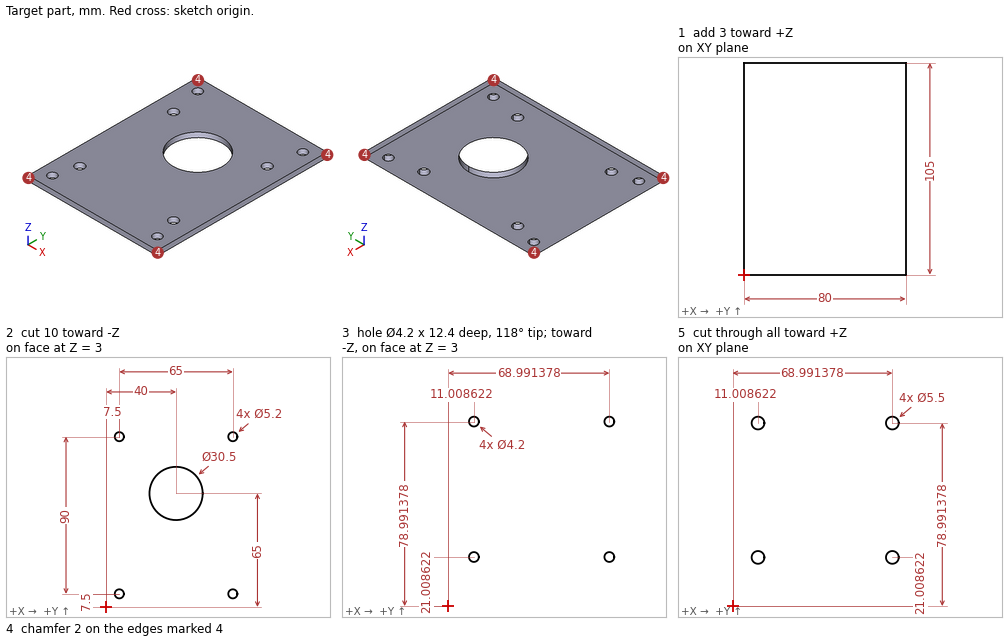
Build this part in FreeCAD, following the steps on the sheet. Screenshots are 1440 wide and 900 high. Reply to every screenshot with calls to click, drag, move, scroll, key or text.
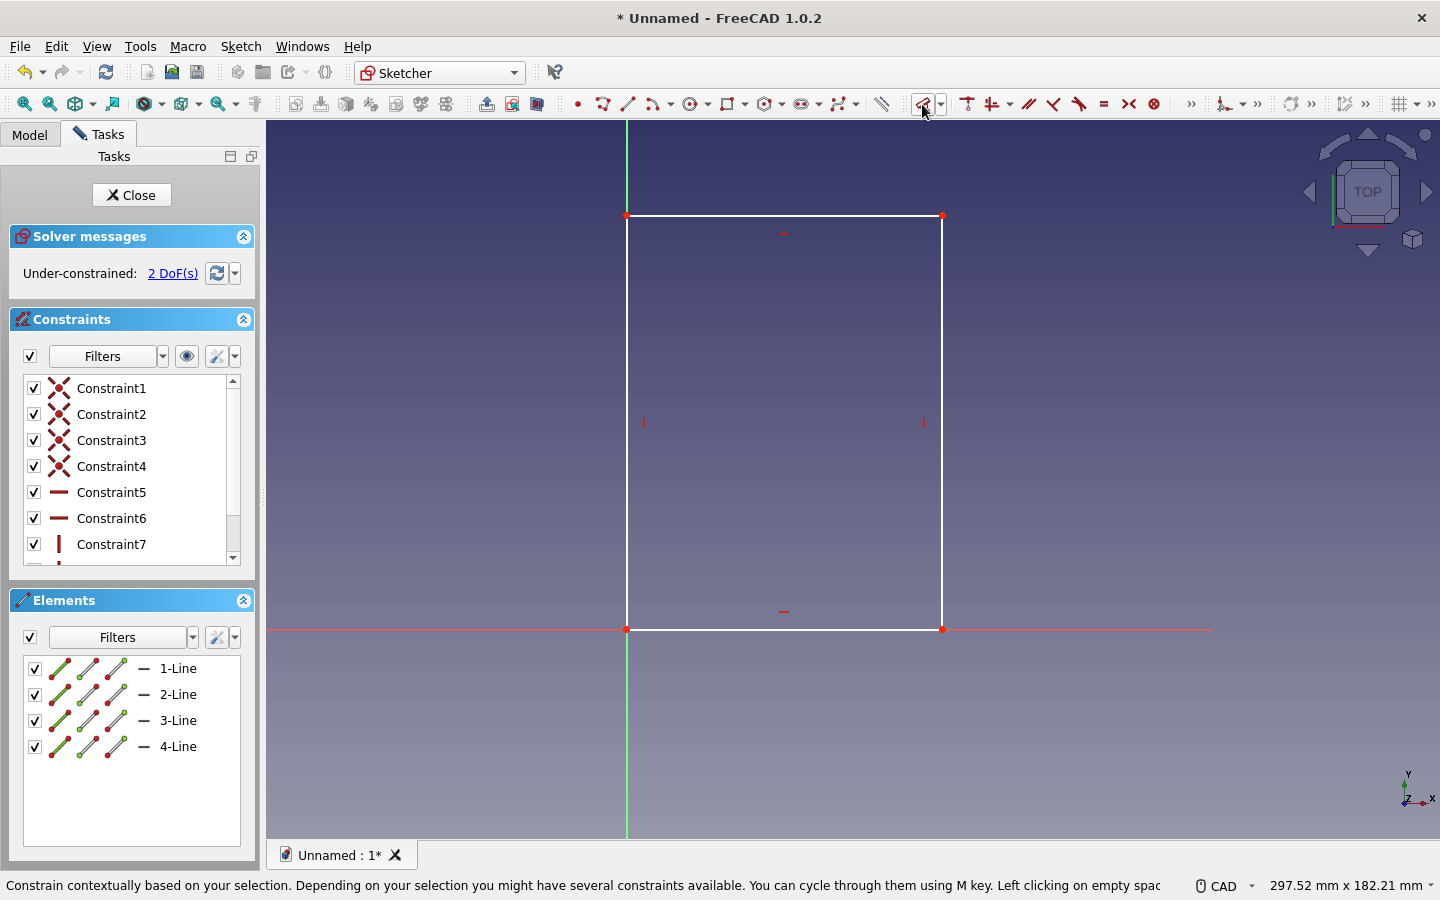
click(721, 630)
click(784, 664)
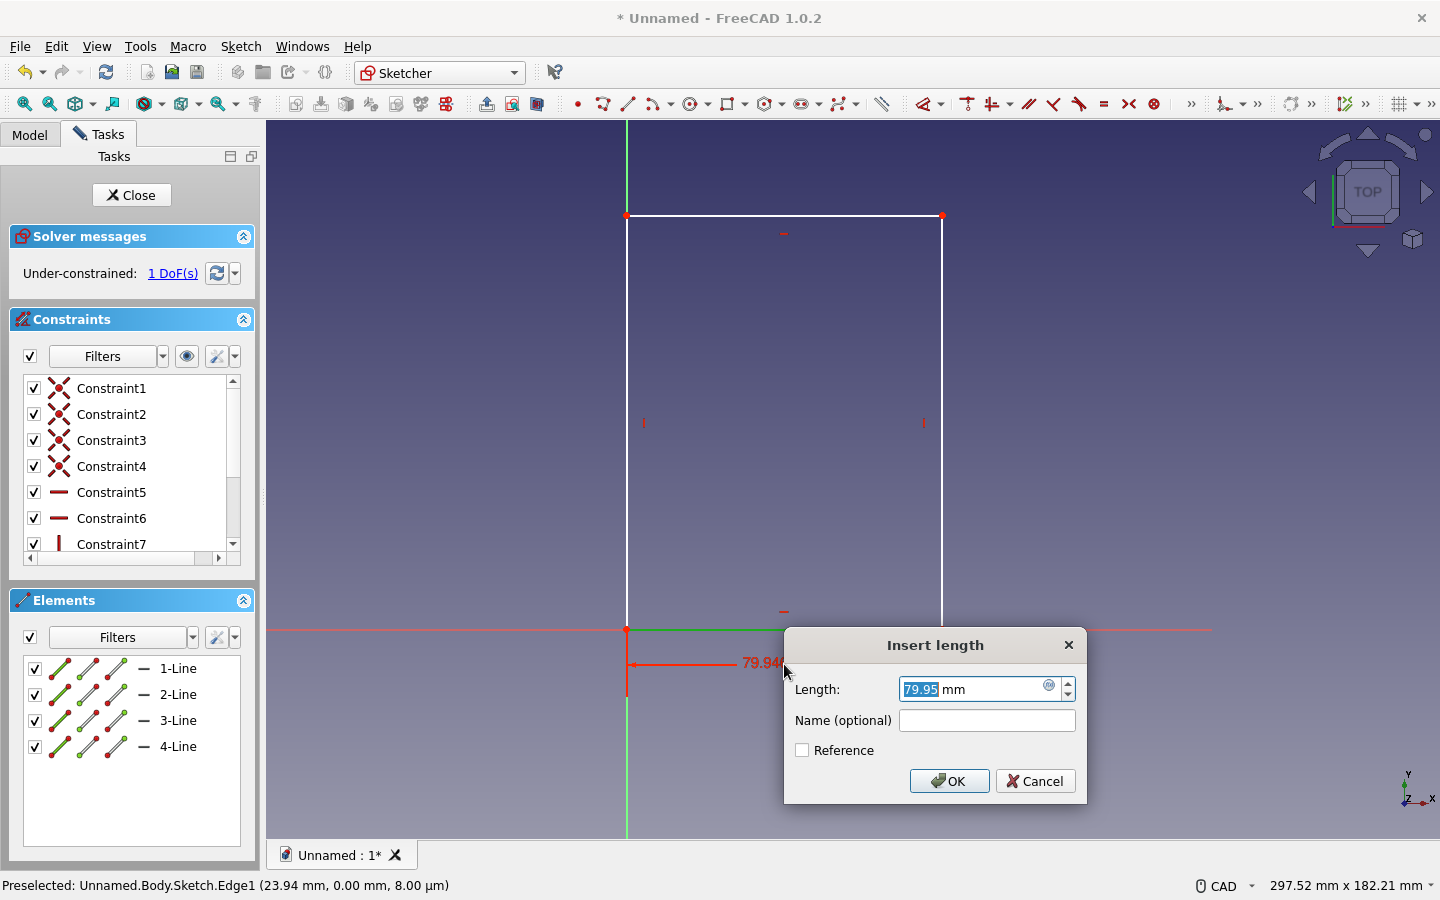
text(80)
key(Return)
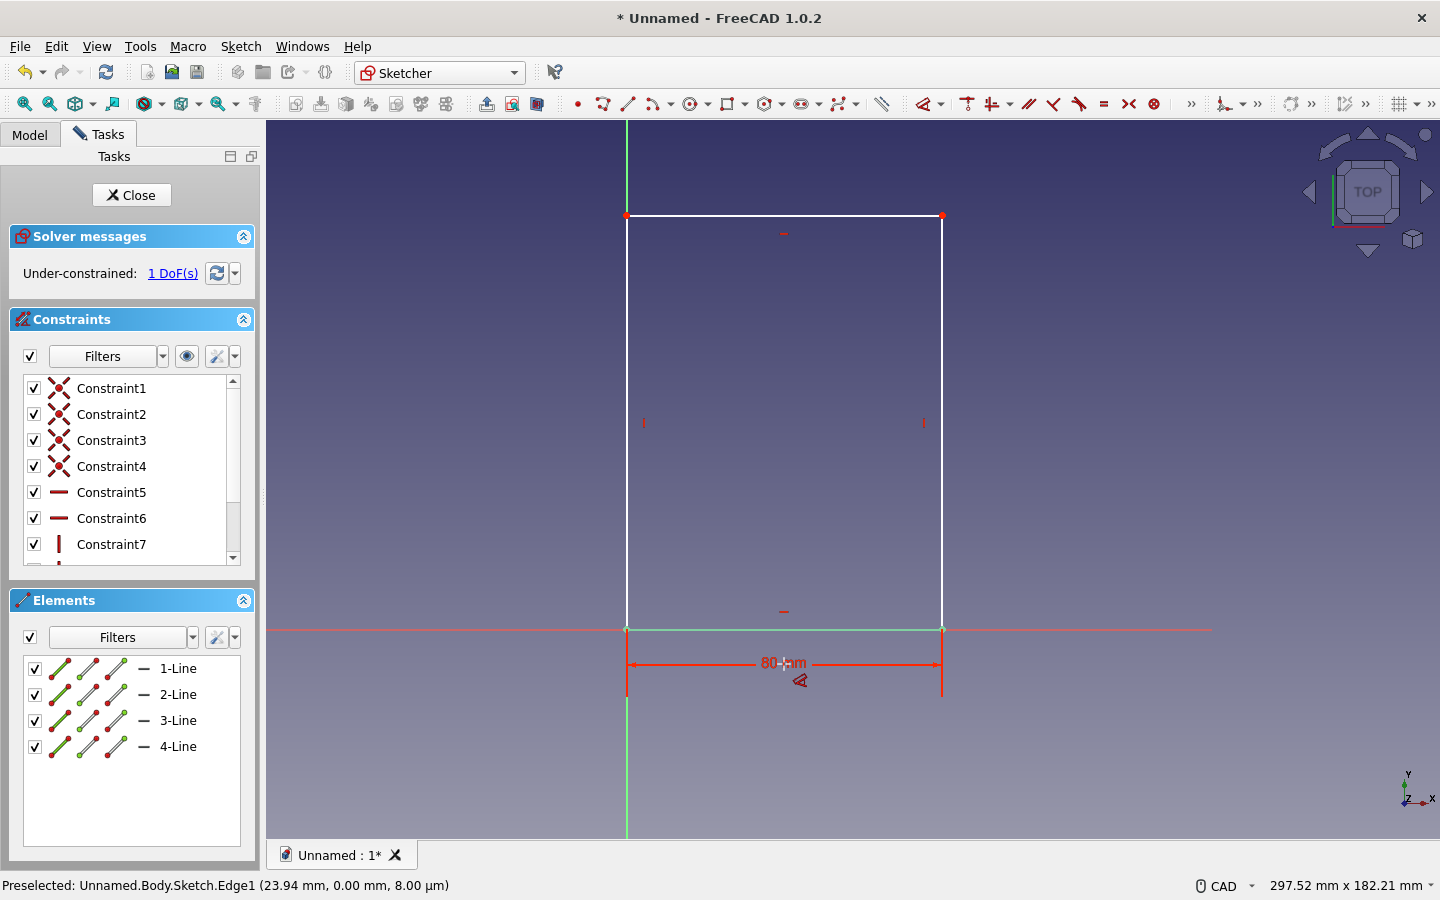
click(942, 505)
click(976, 423)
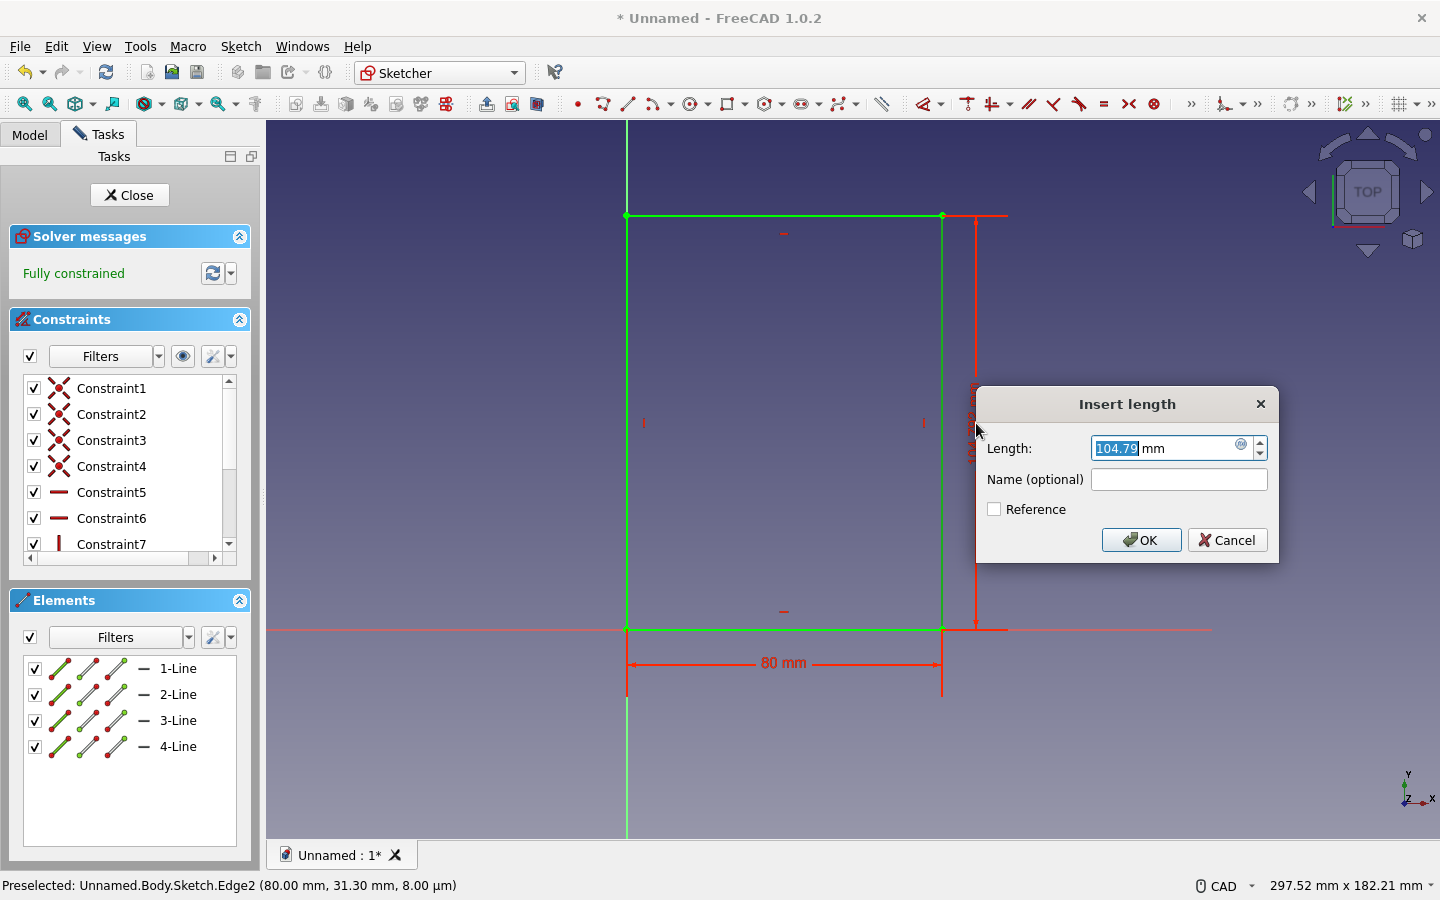
text(105)
key(Return)
key(Escape)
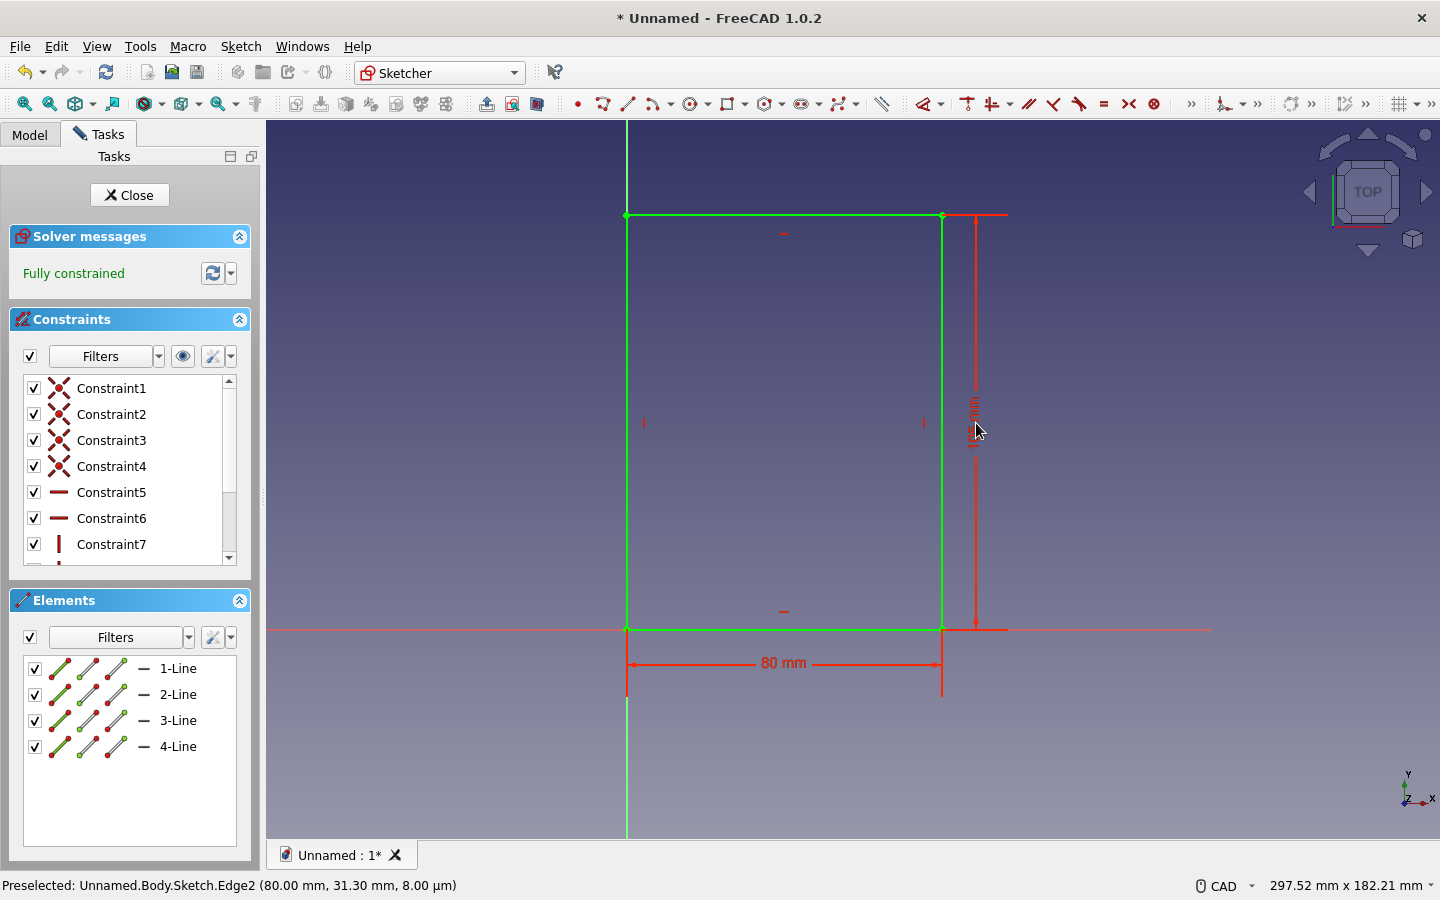
click(130, 195)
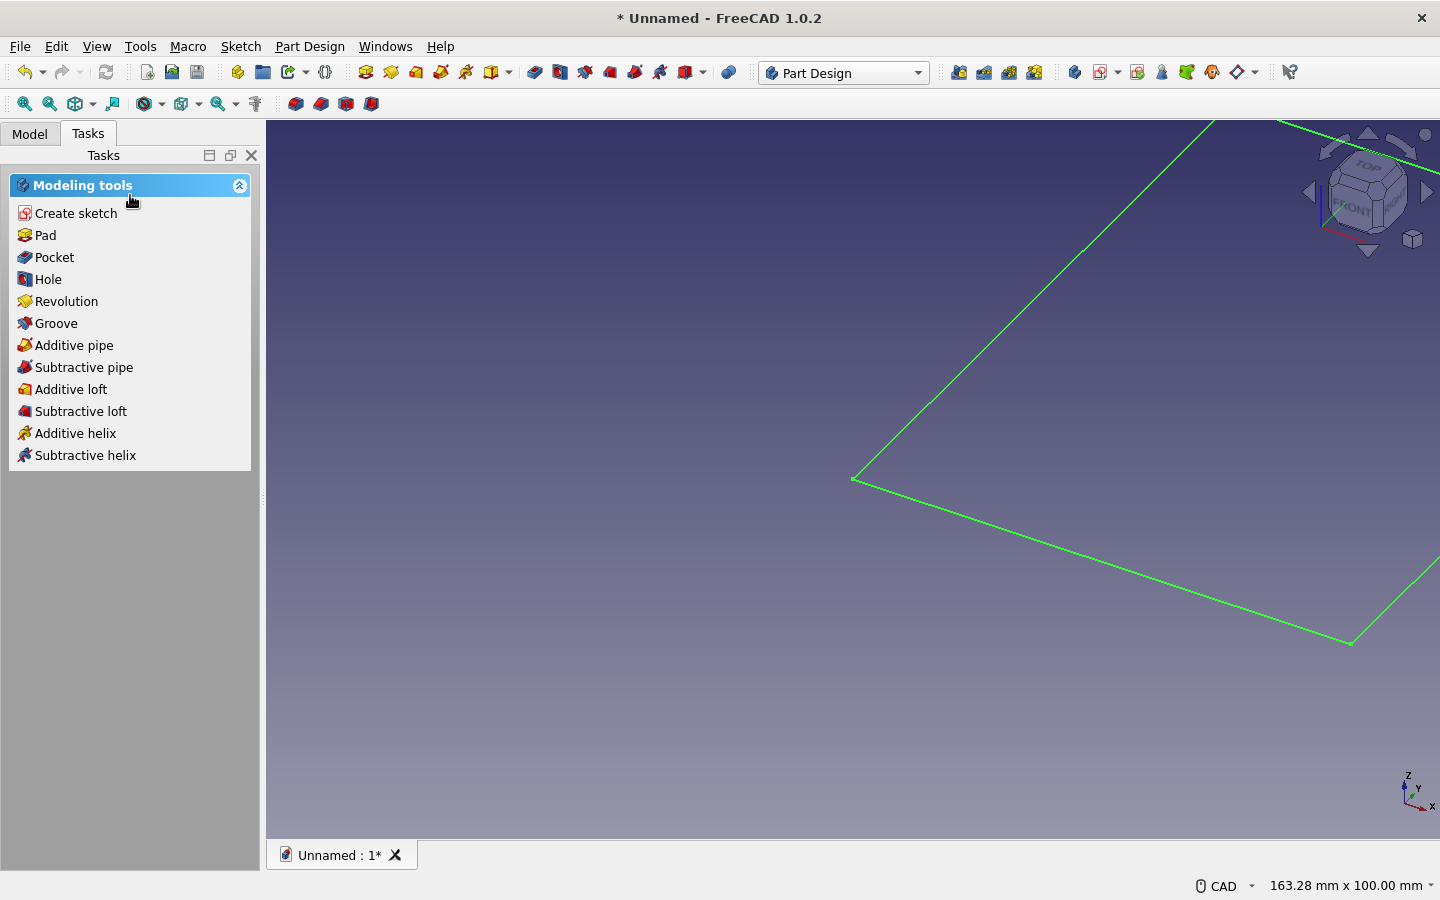
click(366, 72)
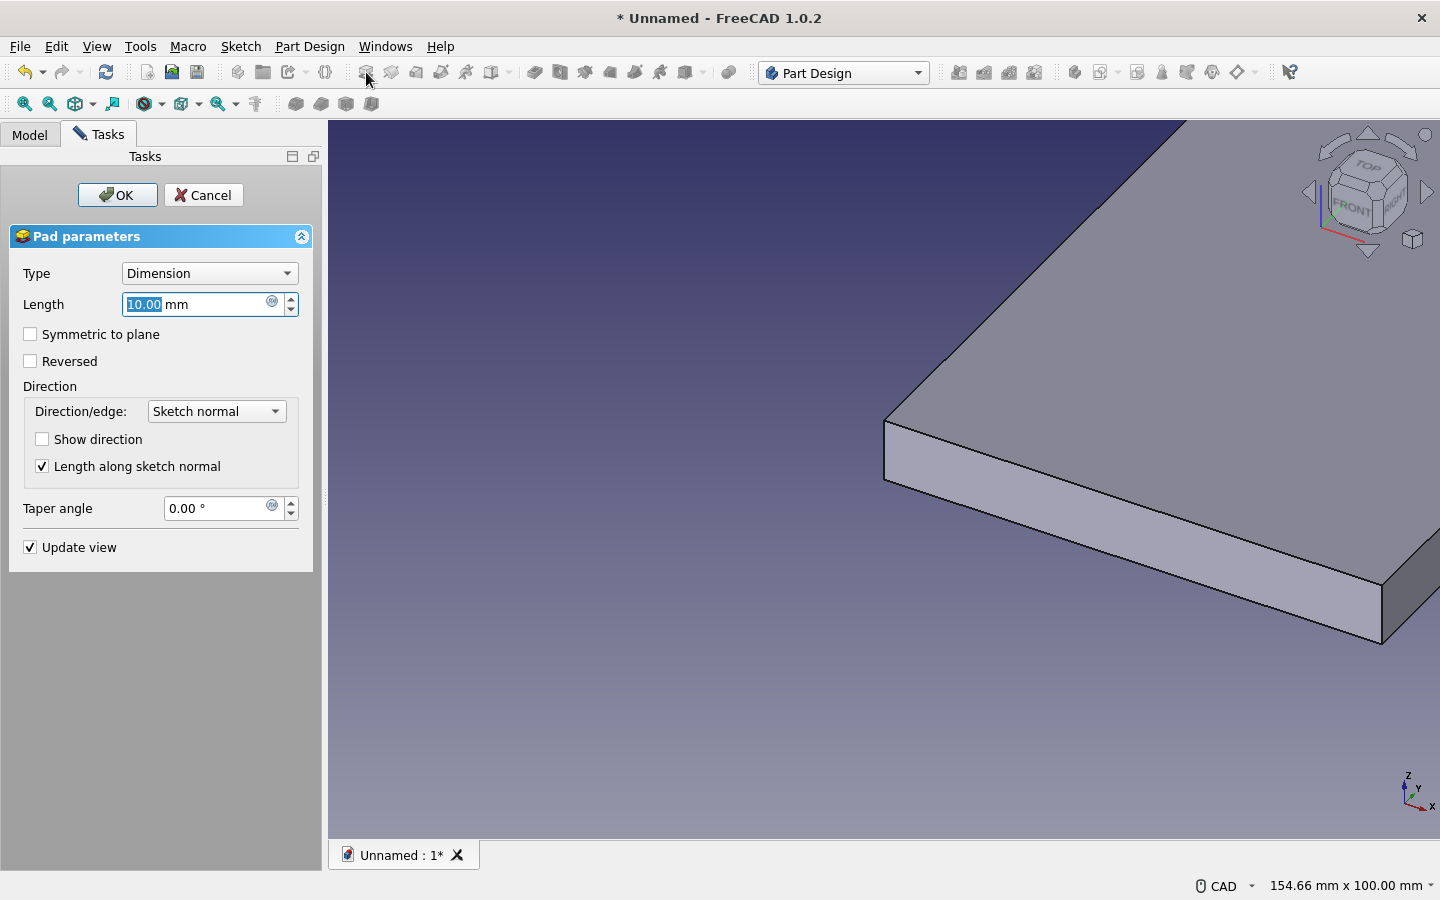
text(3)
key(Tab)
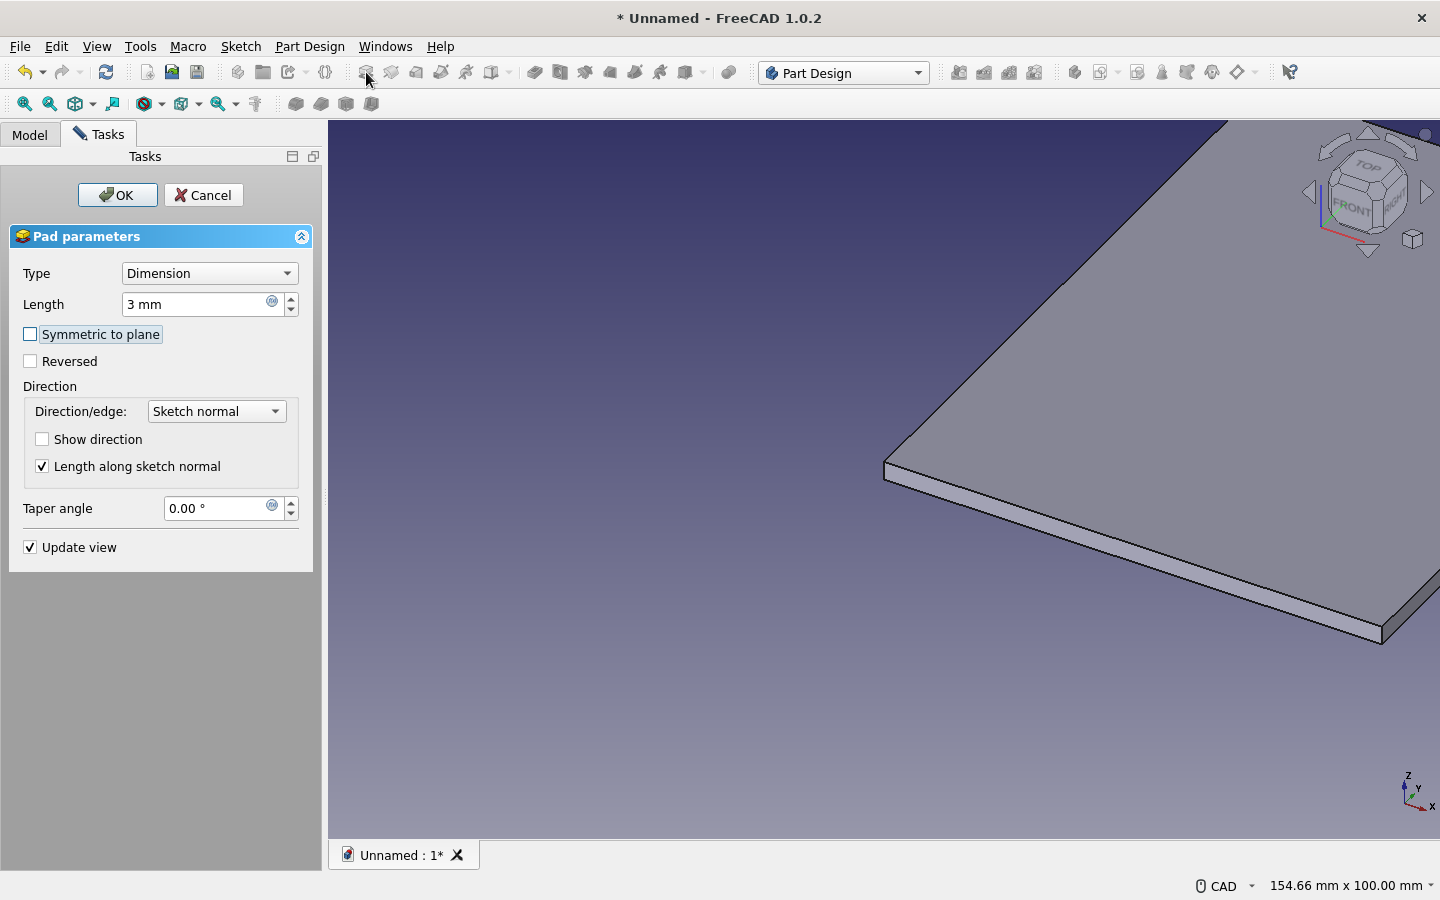
click(118, 195)